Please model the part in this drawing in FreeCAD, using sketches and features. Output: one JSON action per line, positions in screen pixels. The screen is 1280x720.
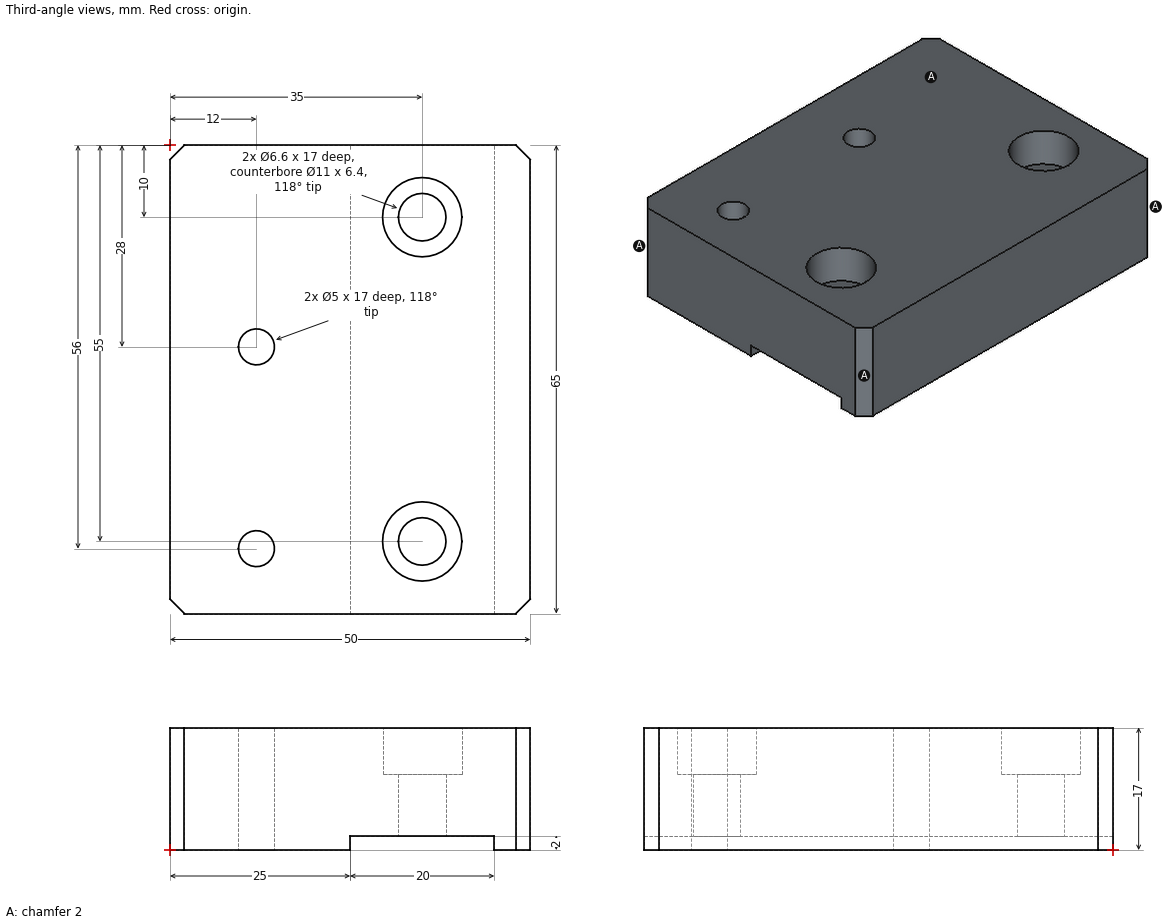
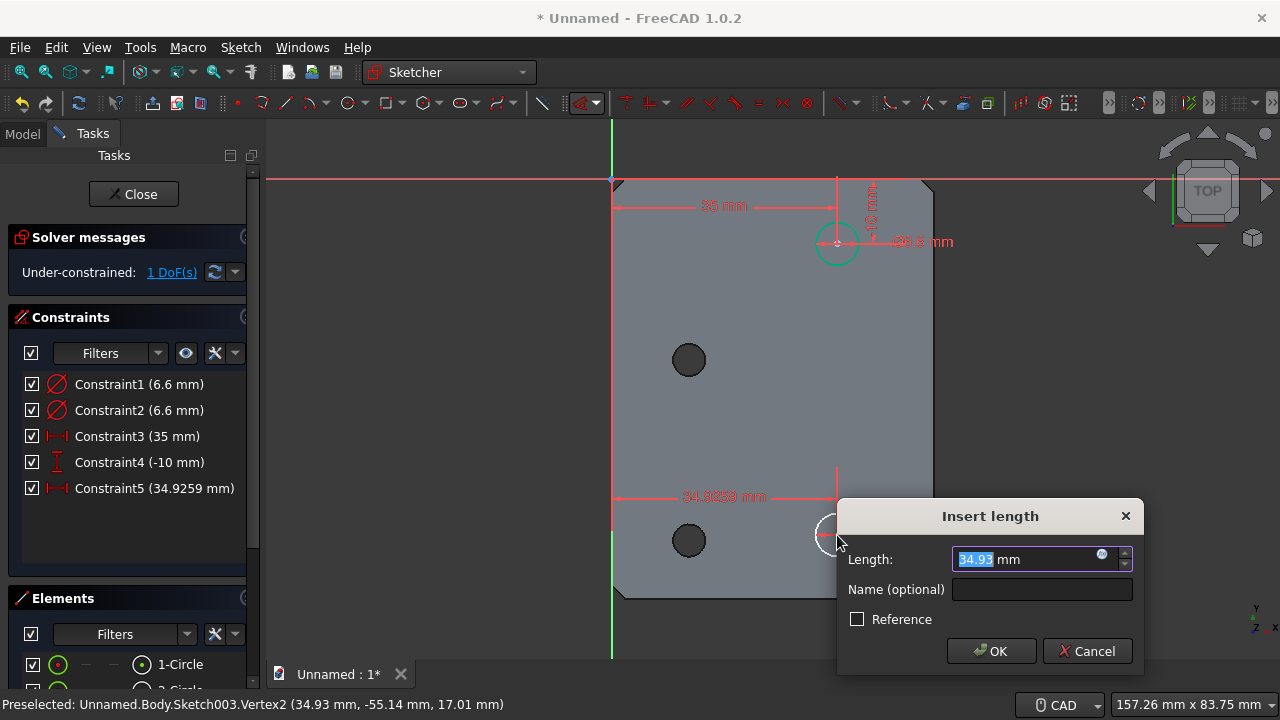
{"action": "type", "text": "35"}
{"action": "key", "text": "Return"}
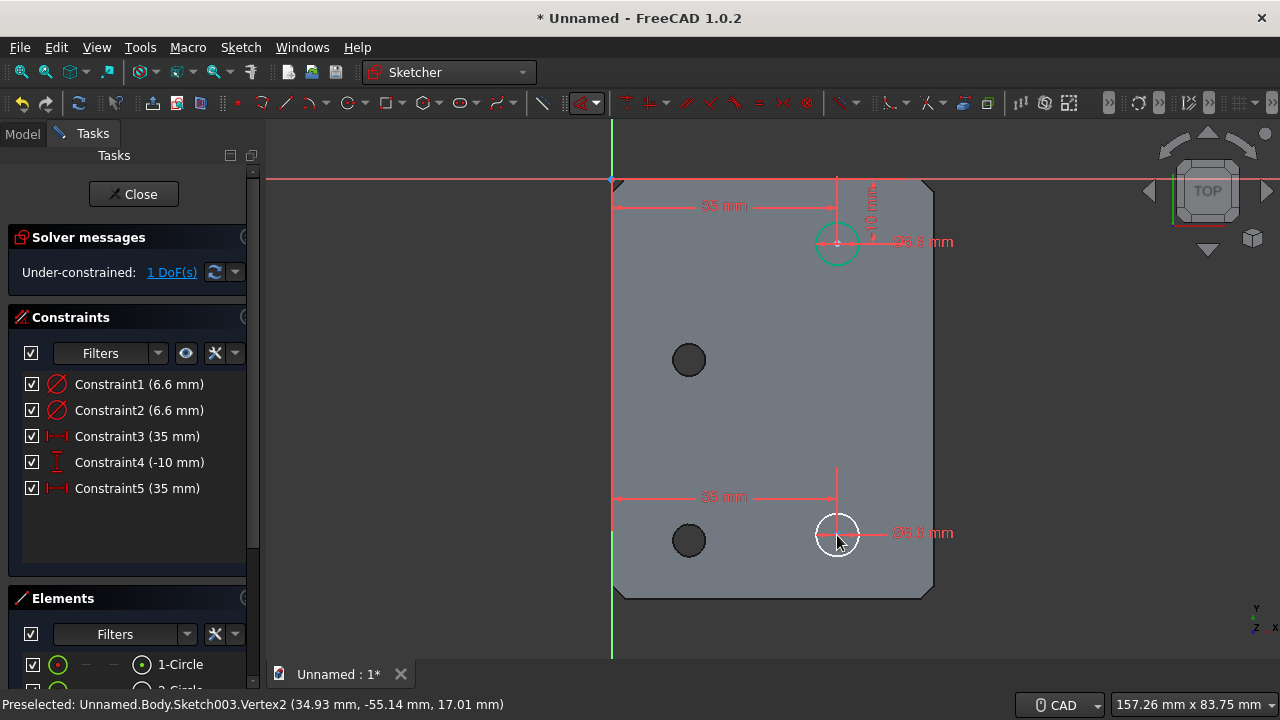
{"action": "left_click", "coordinate": [837, 535]}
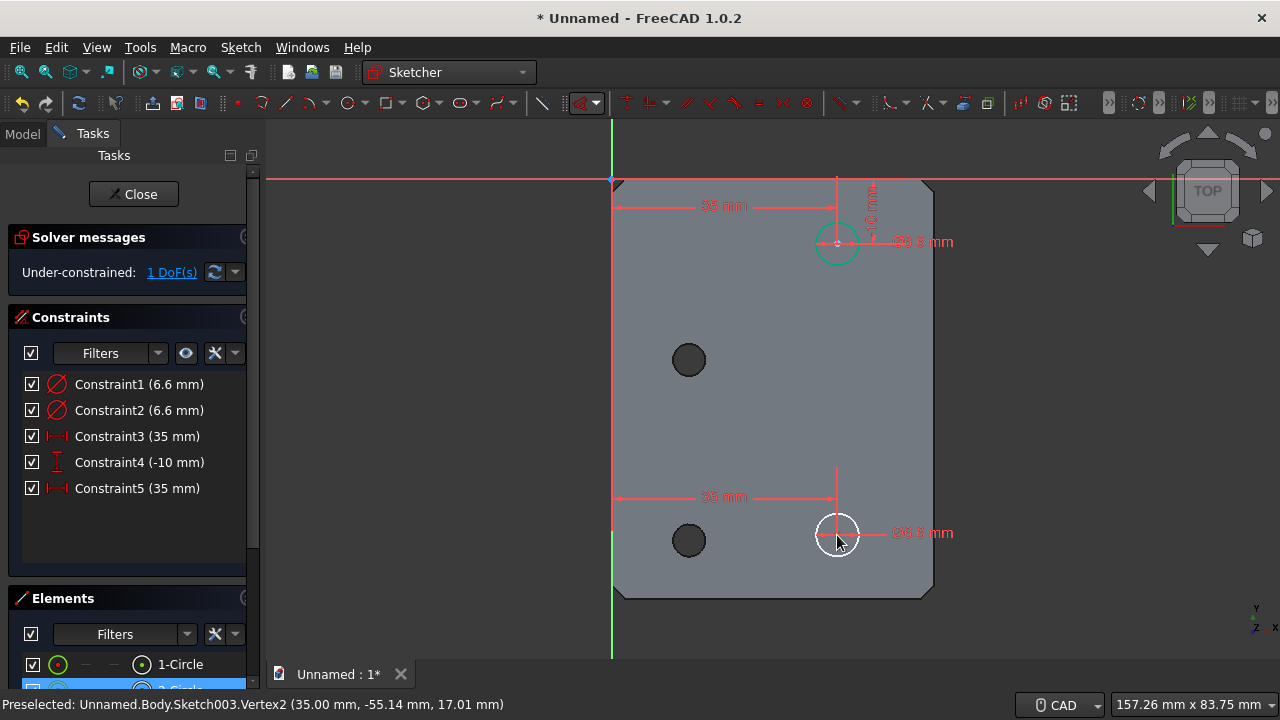
{"action": "left_click", "coordinate": [598, 104]}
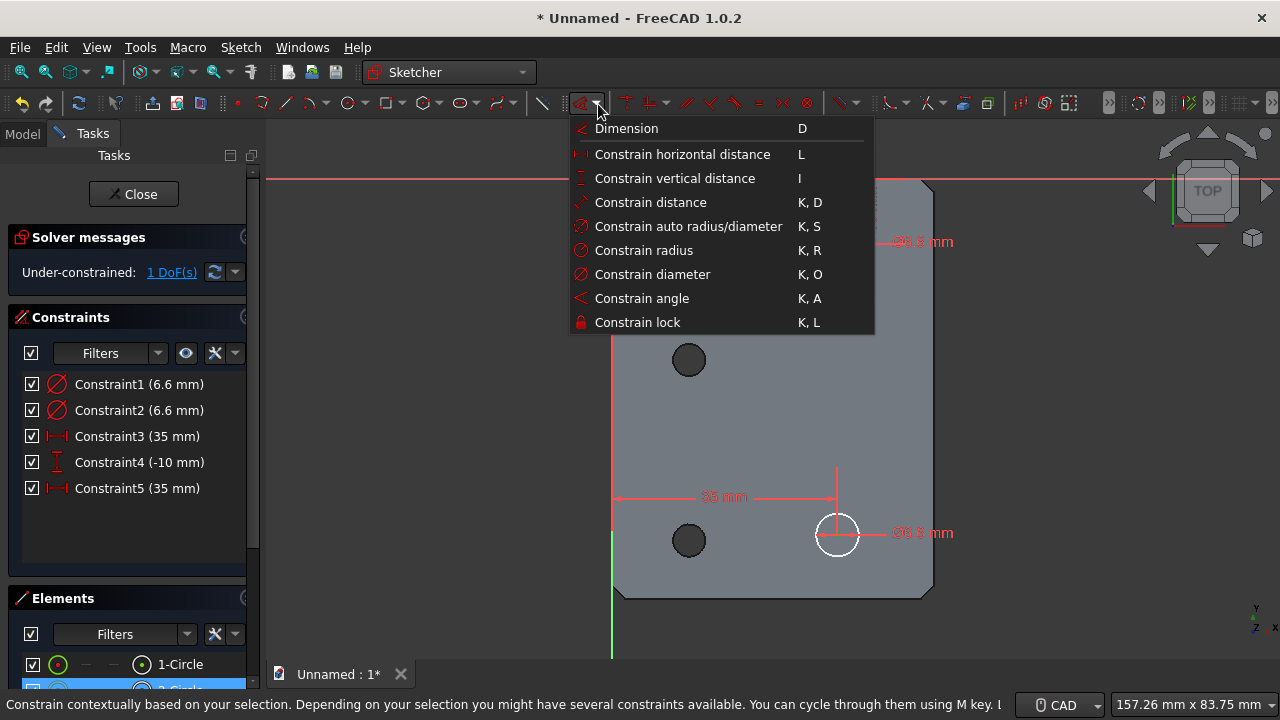
{"action": "left_click", "coordinate": [722, 178]}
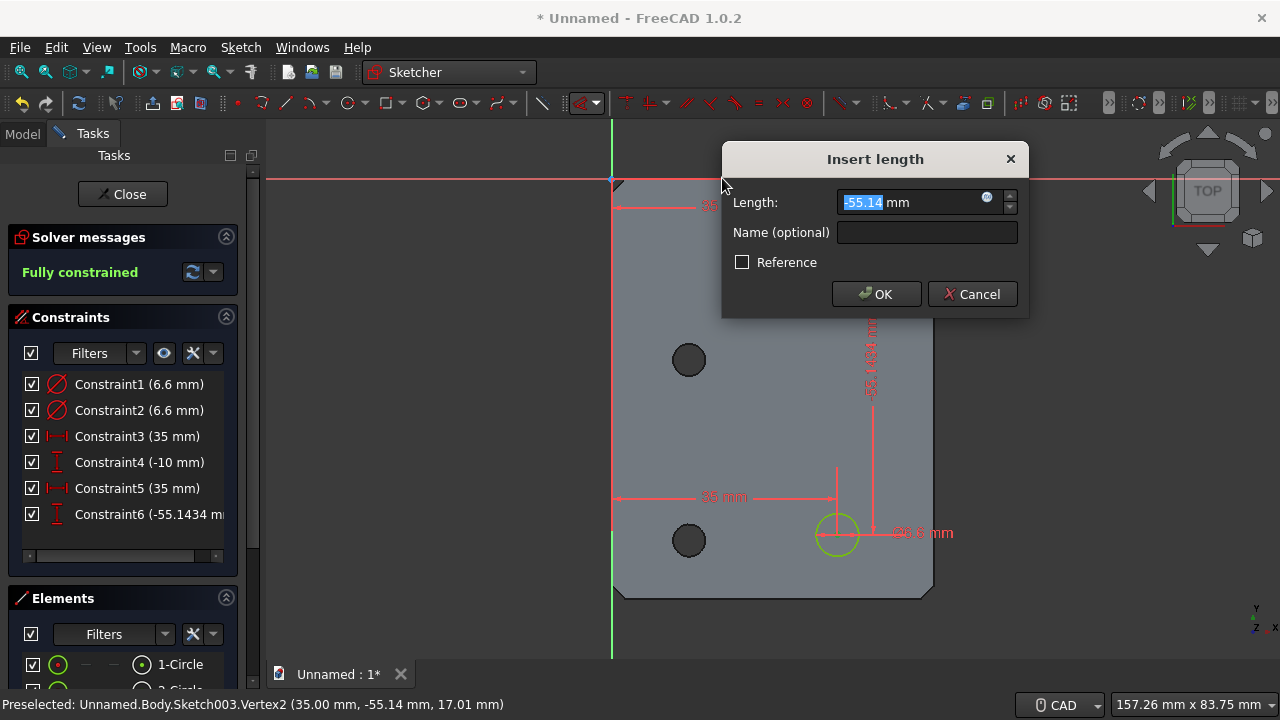
{"action": "type", "text": "-55"}
{"action": "key", "text": "Return"}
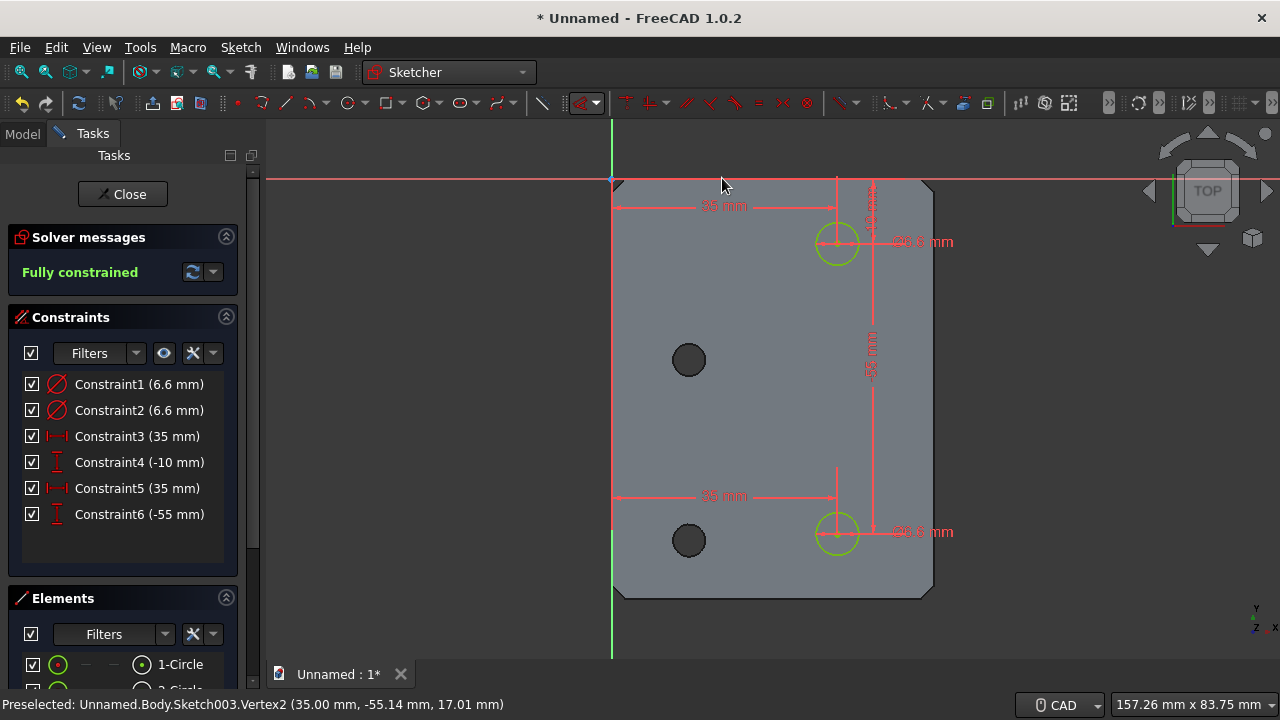
{"action": "left_click", "coordinate": [123, 194]}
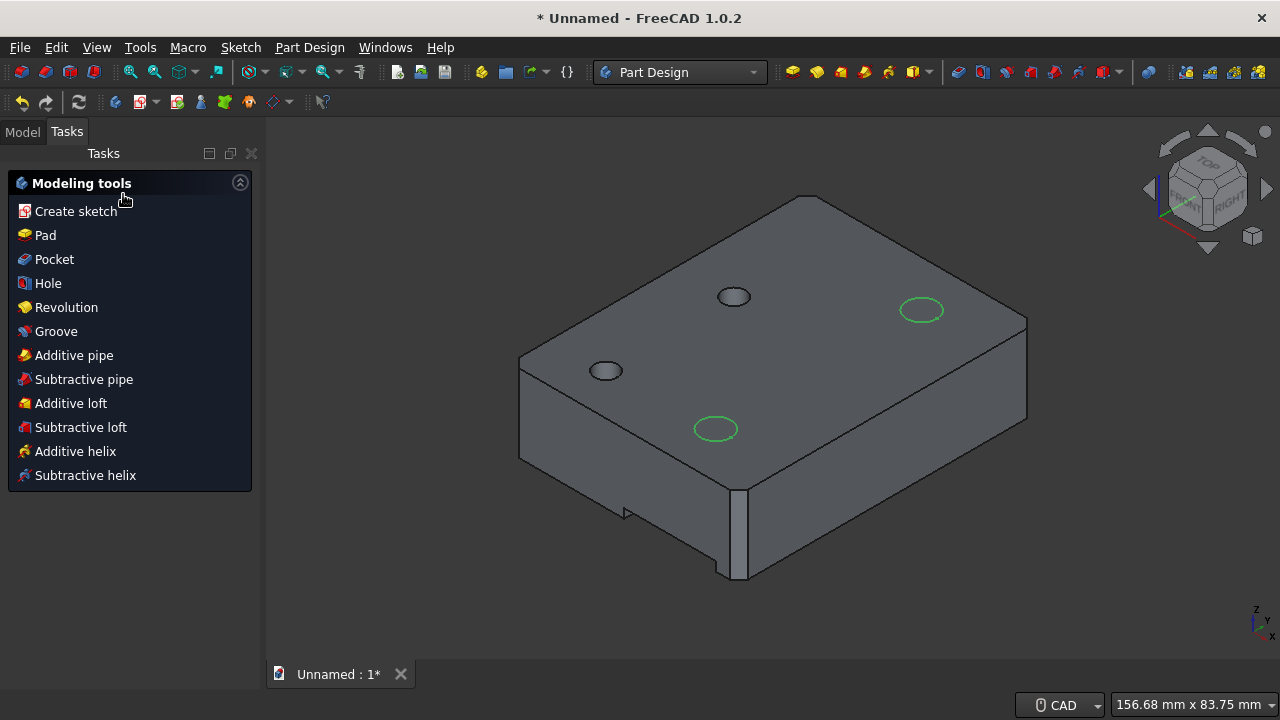
{"action": "left_click", "coordinate": [984, 72]}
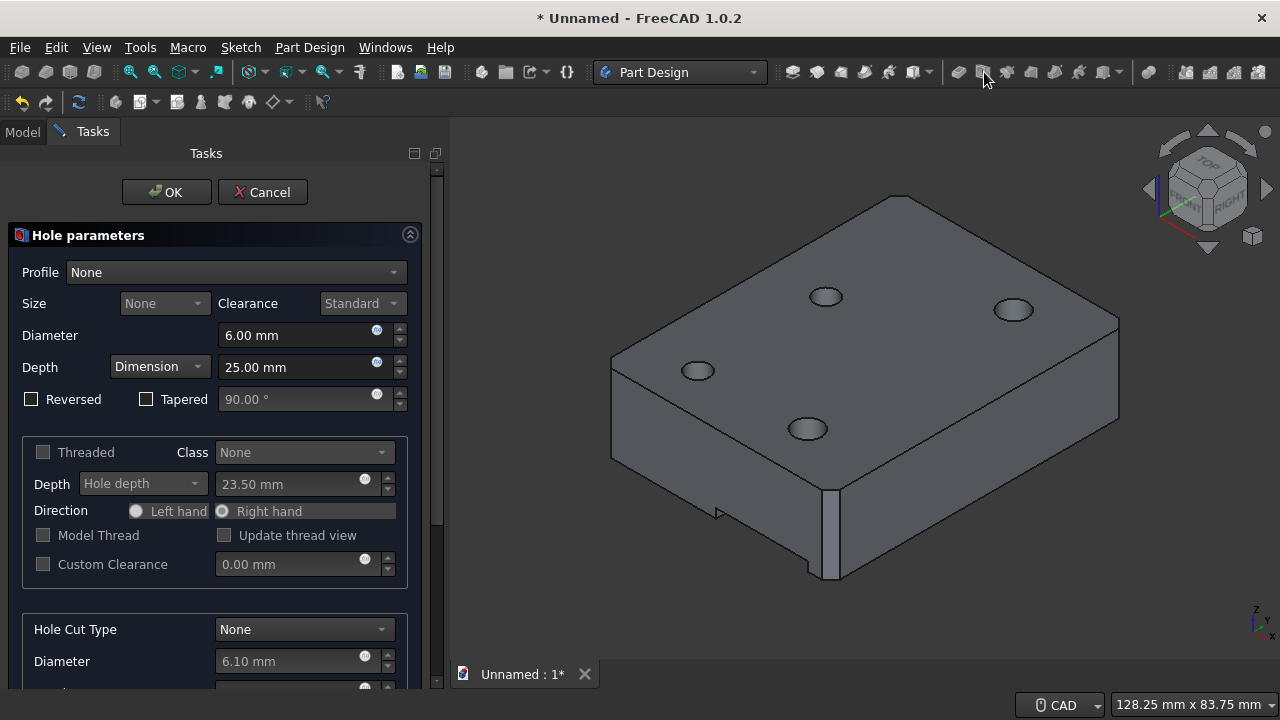
{"action": "triple_click", "coordinate": [305, 335]}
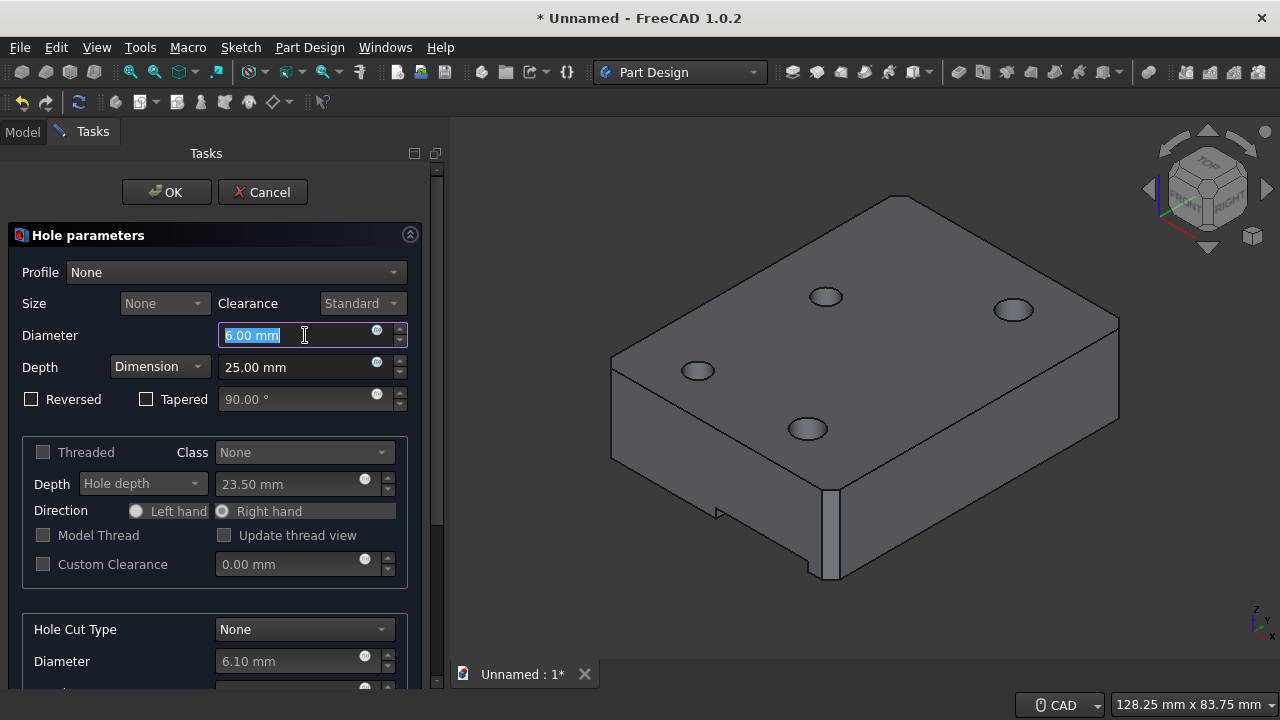
{"action": "type", "text": "6.6"}
{"action": "key", "text": "Tab"}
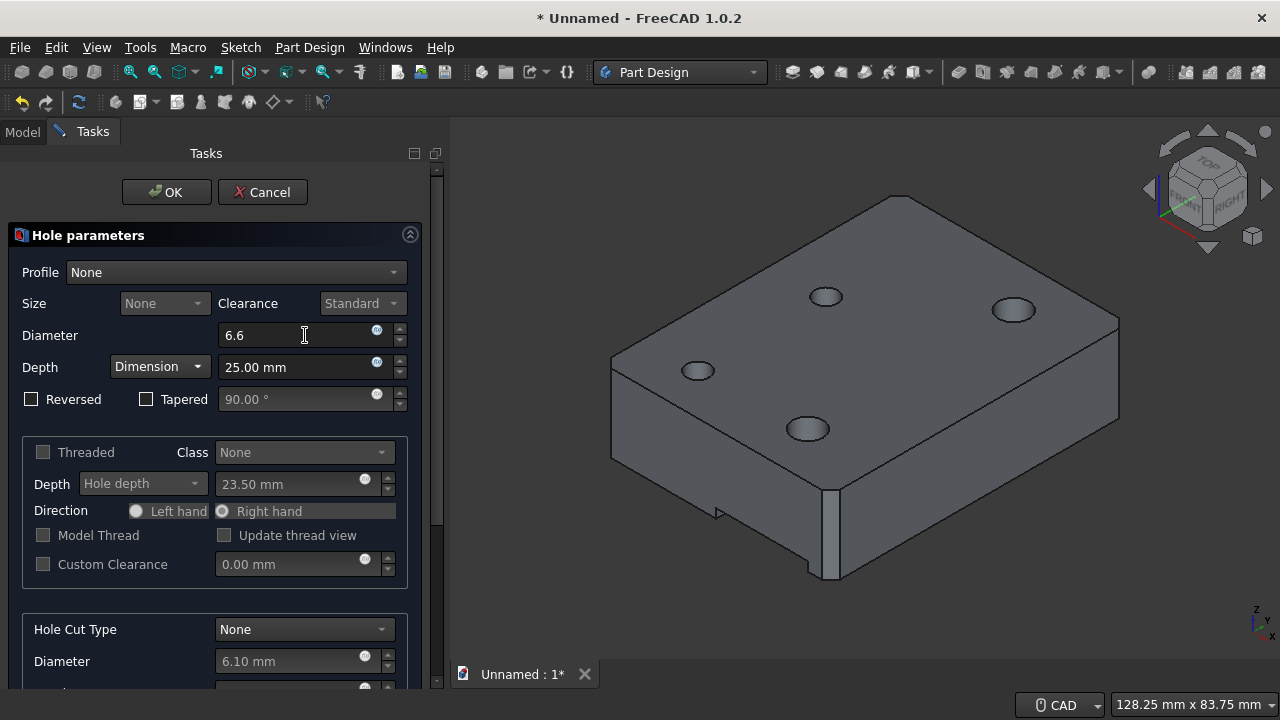
{"action": "triple_click", "coordinate": [305, 367]}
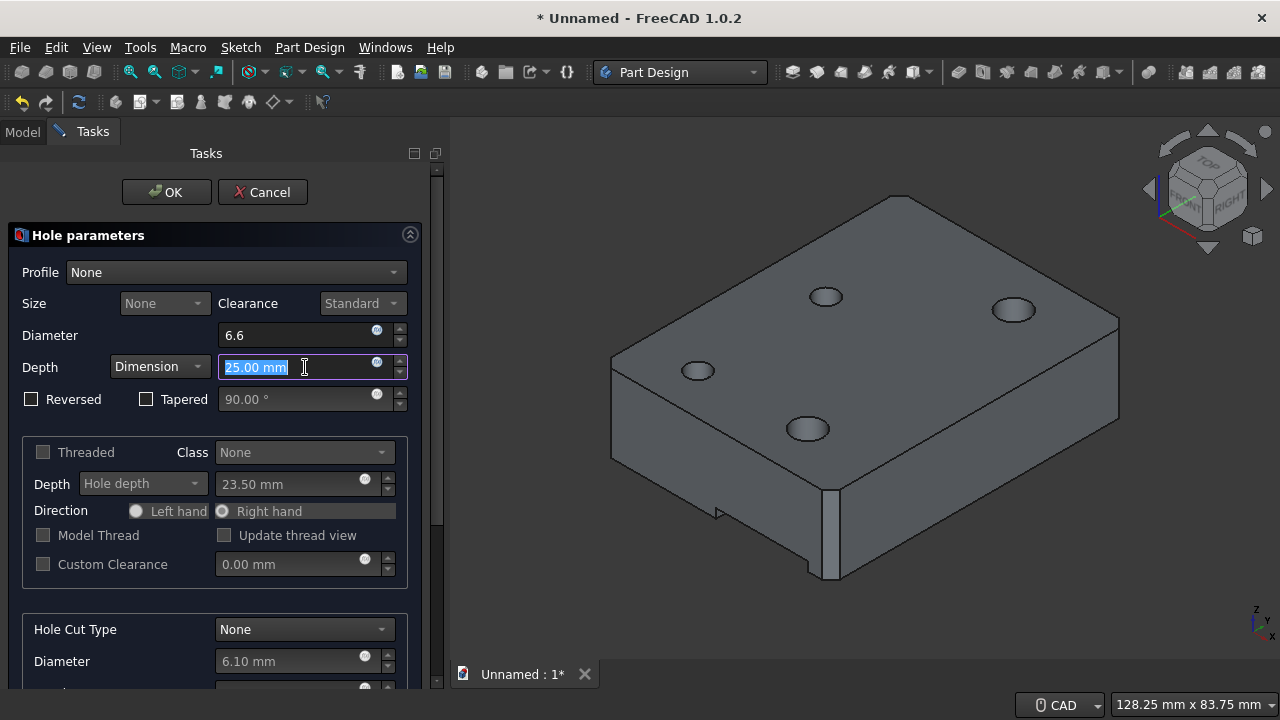
{"action": "type", "text": "17"}
{"action": "key", "text": "Tab"}